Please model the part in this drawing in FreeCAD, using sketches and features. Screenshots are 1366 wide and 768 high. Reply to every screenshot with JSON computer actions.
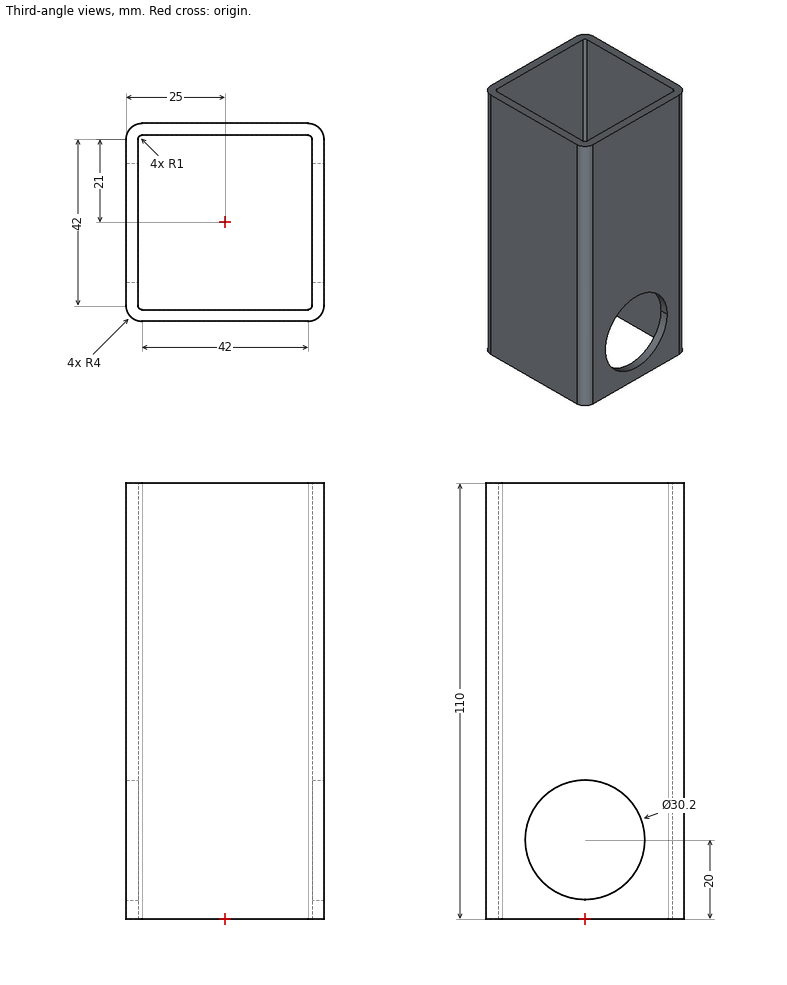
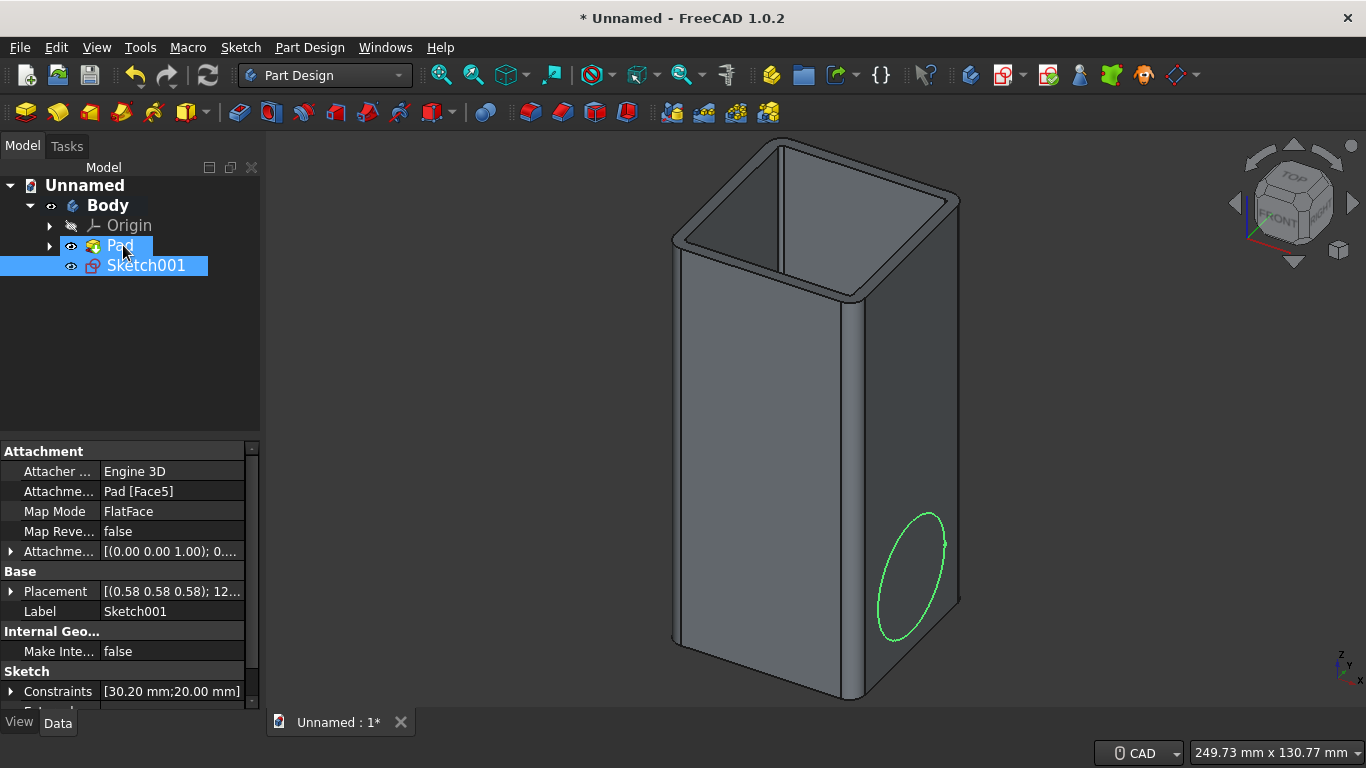
{"action": "left_click", "coordinate": [240, 112]}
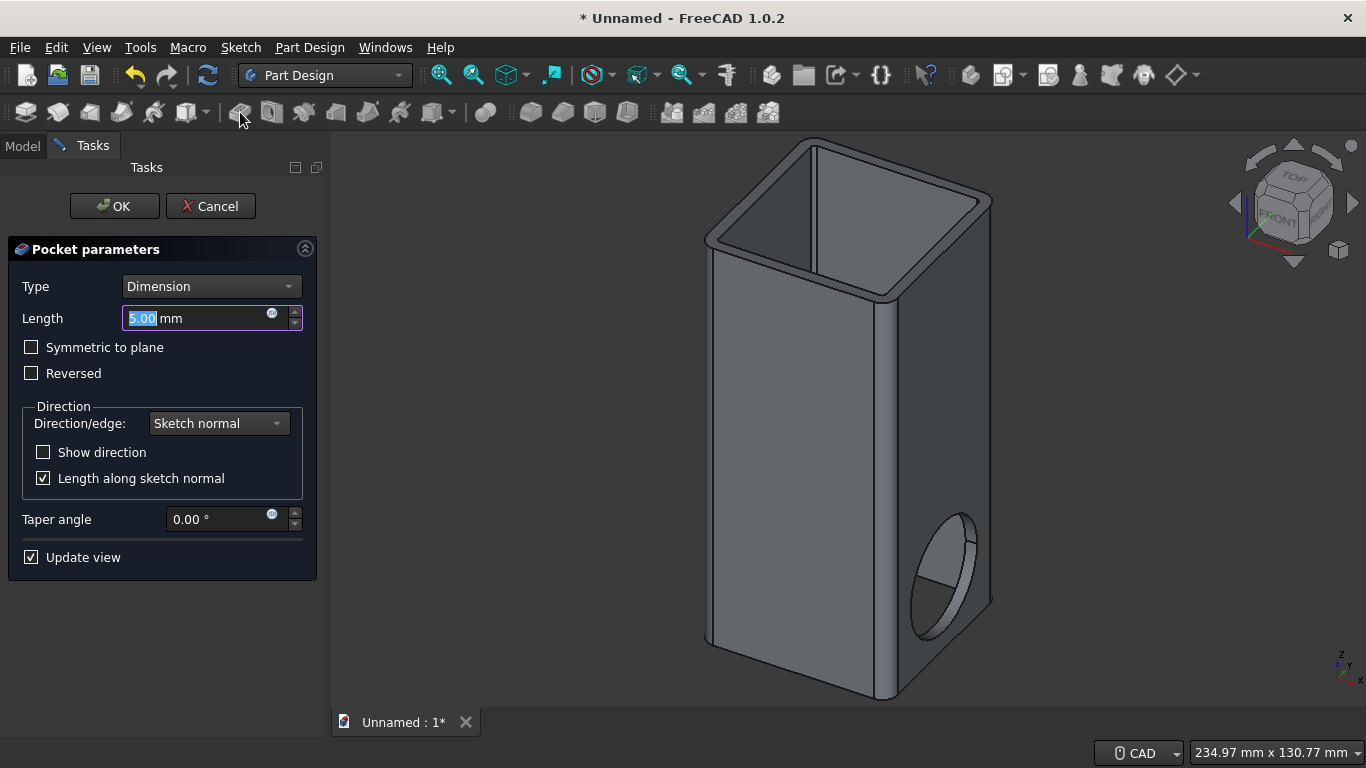
{"action": "left_click", "coordinate": [212, 286]}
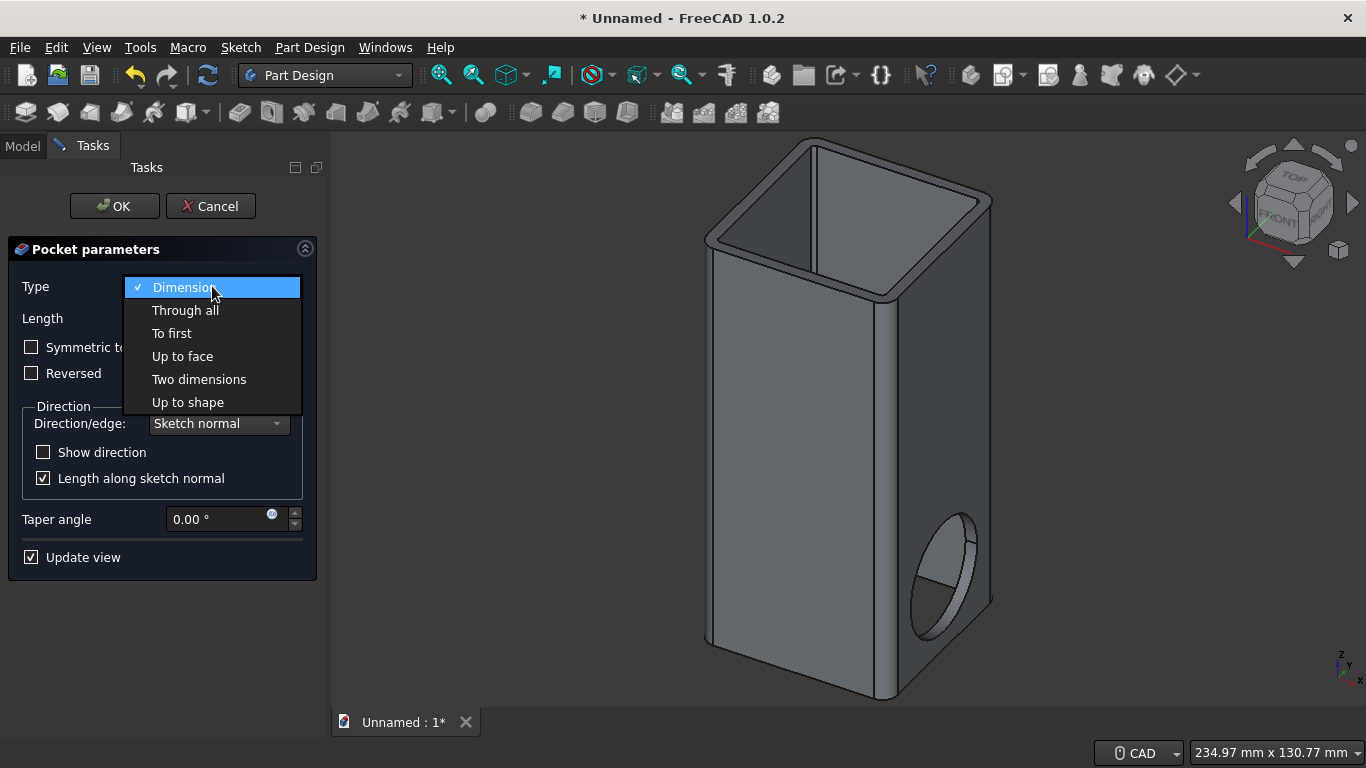
{"action": "left_click", "coordinate": [212, 310]}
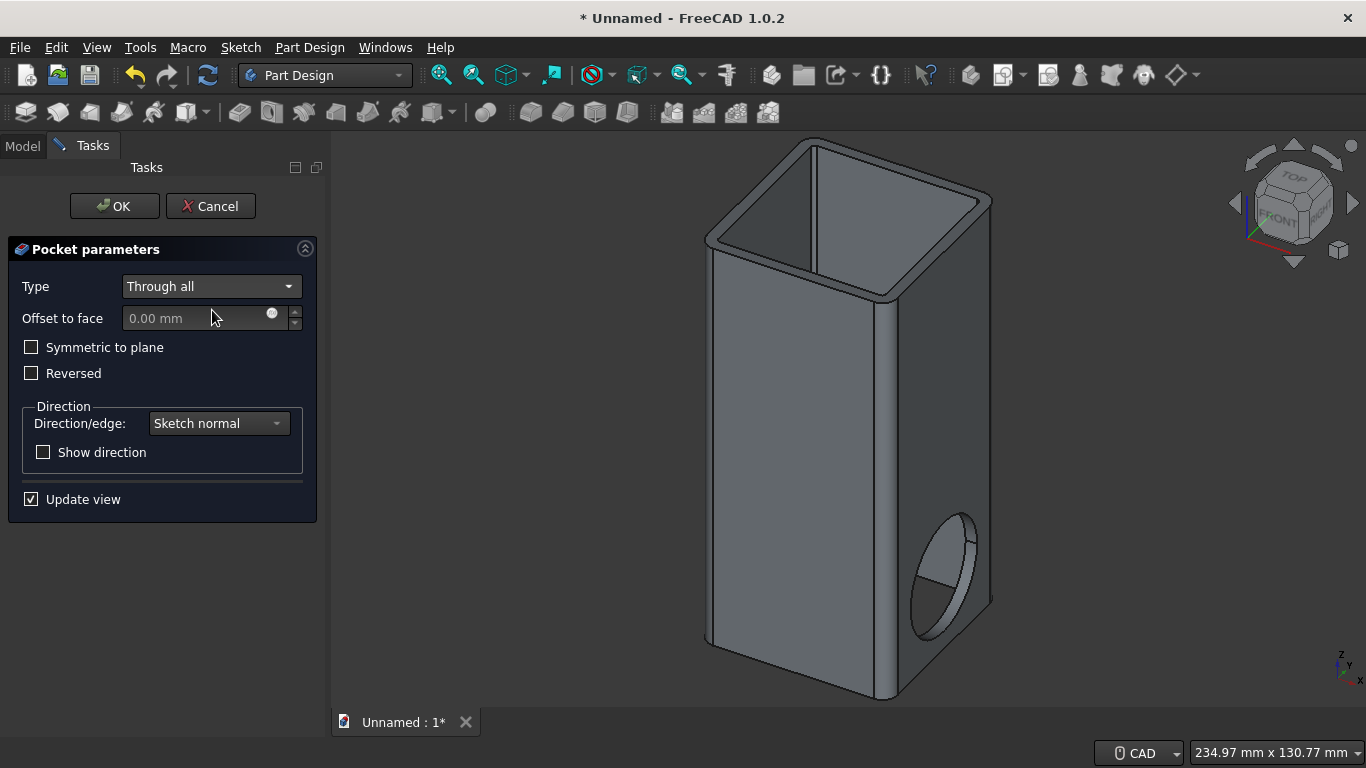
{"action": "left_click", "coordinate": [115, 206]}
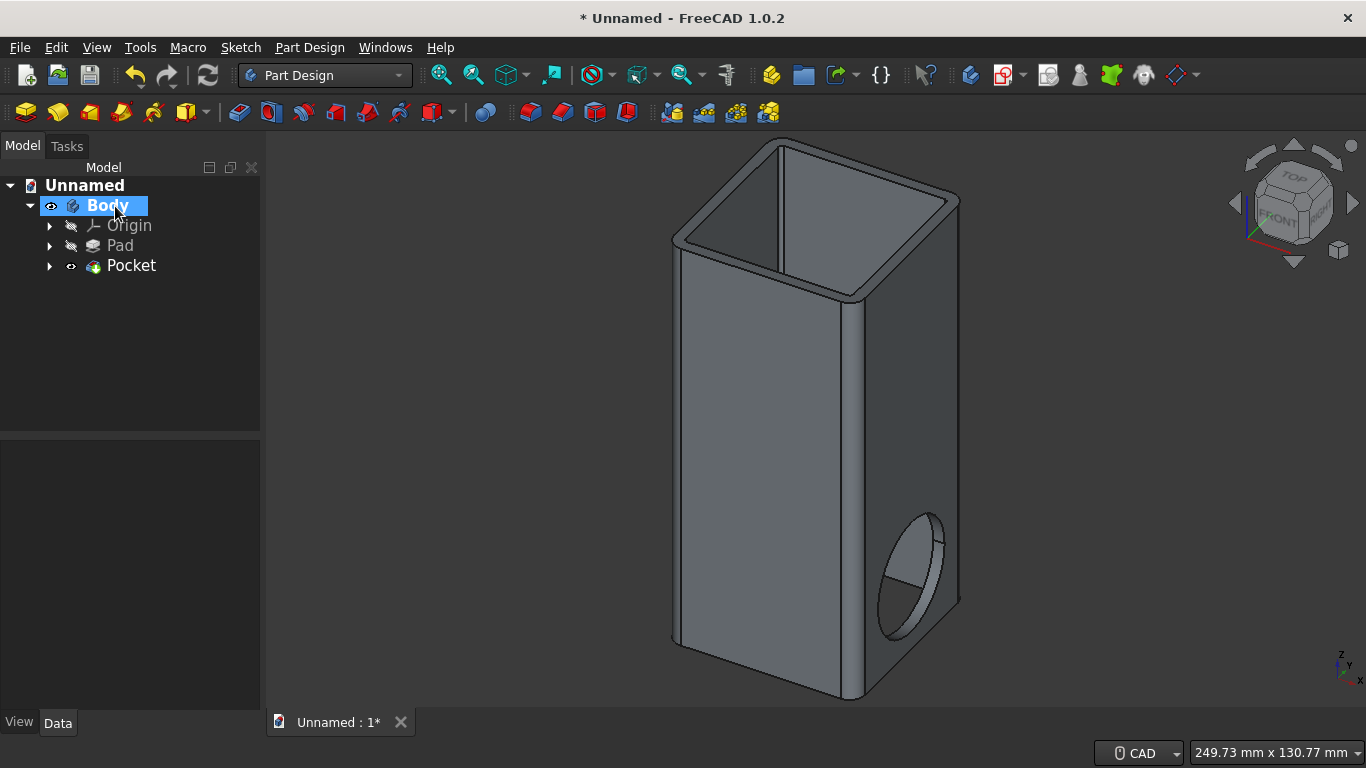
{"action": "key", "text": "0"}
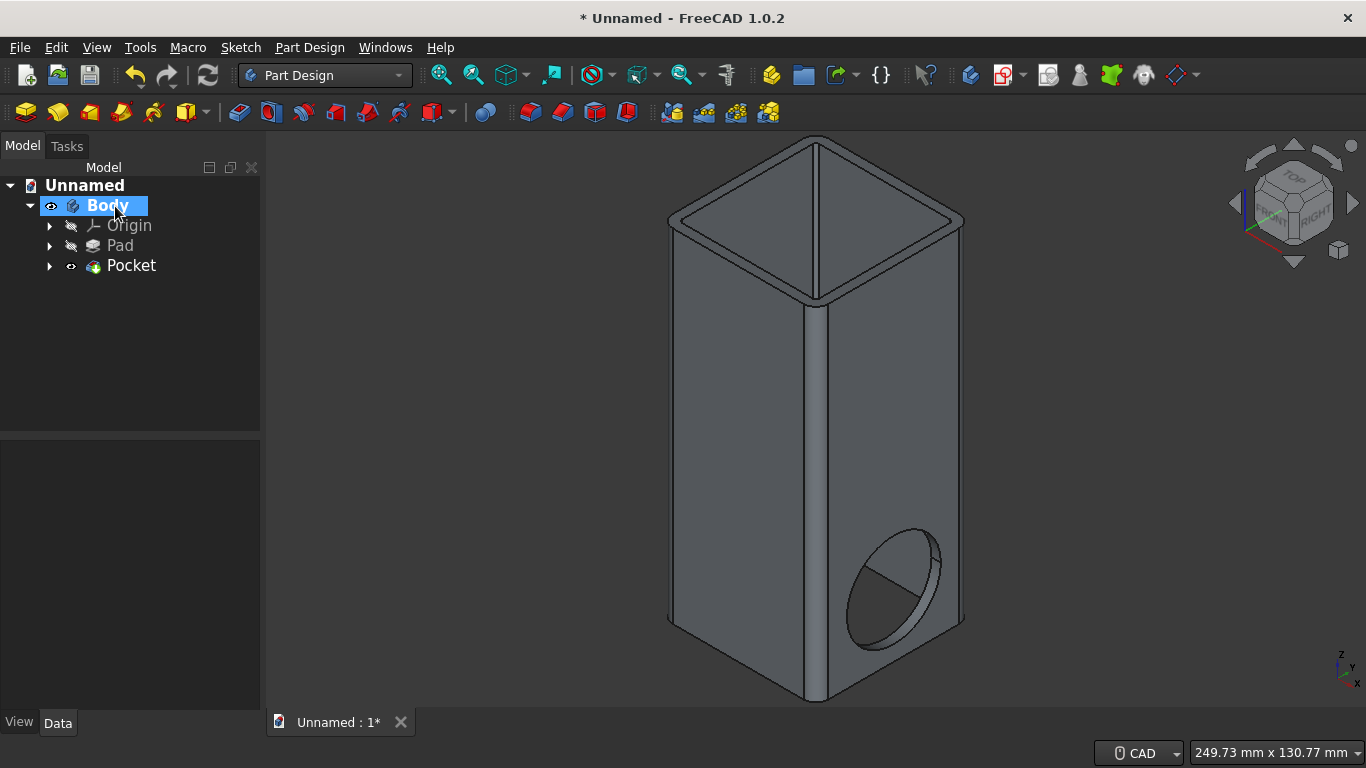
{"action": "left_click", "coordinate": [442, 76]}